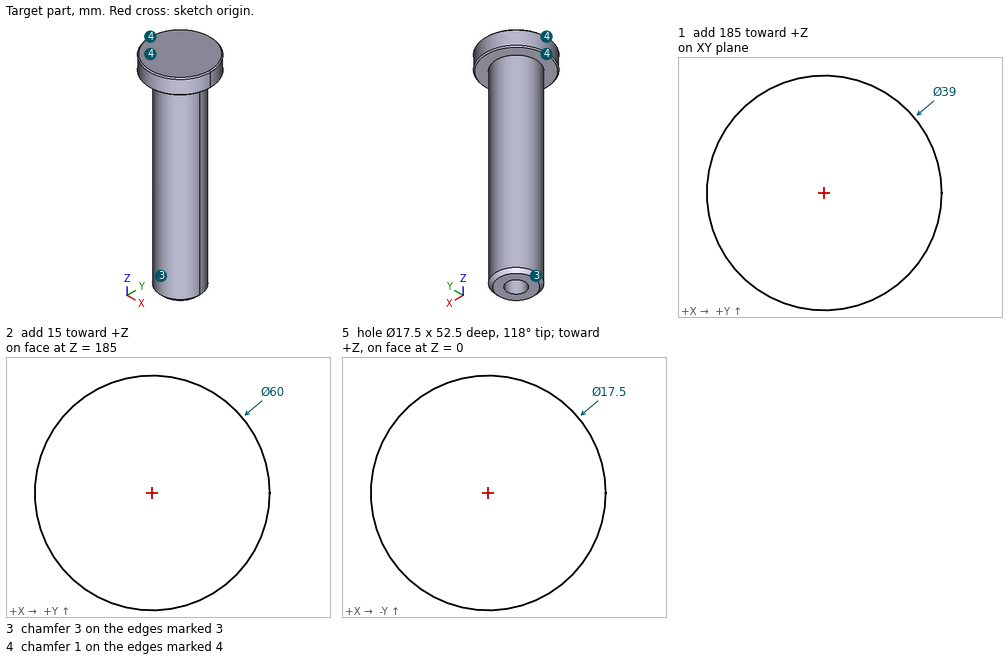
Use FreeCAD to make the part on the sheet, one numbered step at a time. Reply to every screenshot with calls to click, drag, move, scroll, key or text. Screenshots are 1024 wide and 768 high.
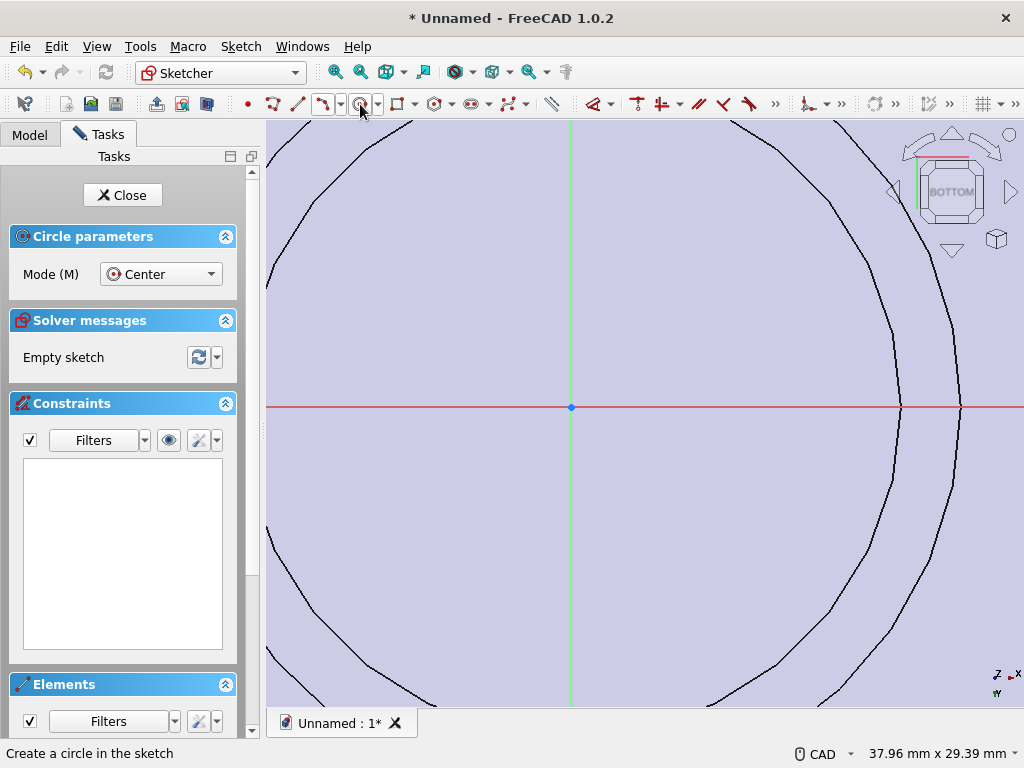
click(571, 407)
click(695, 284)
key(Escape)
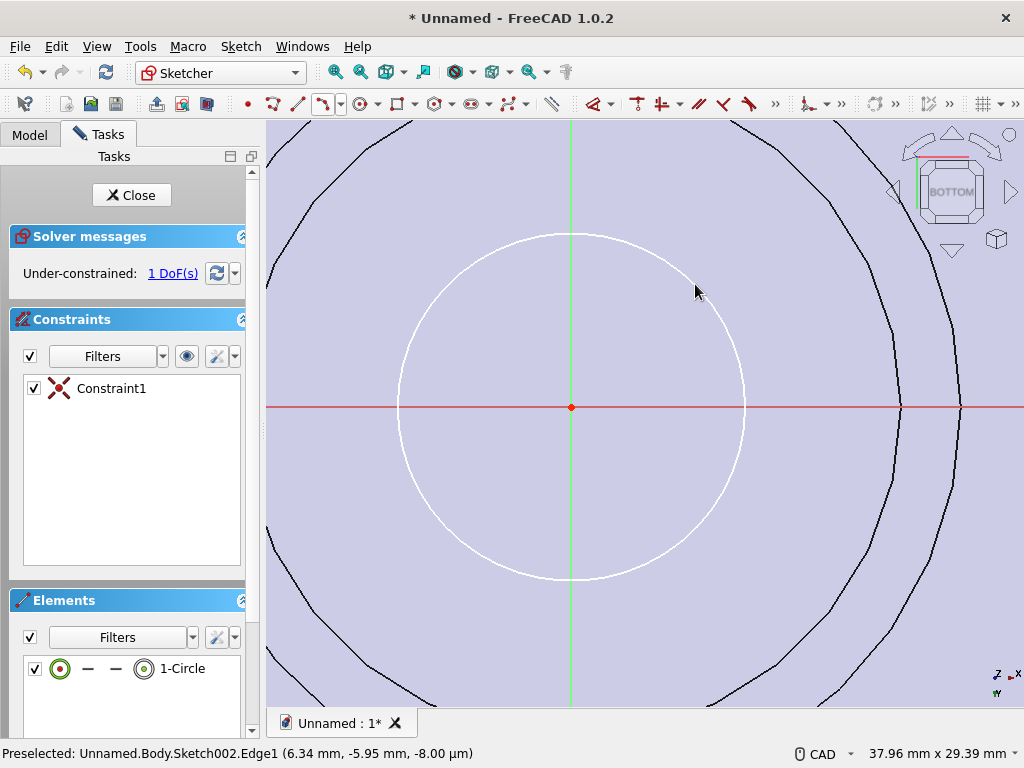
click(592, 104)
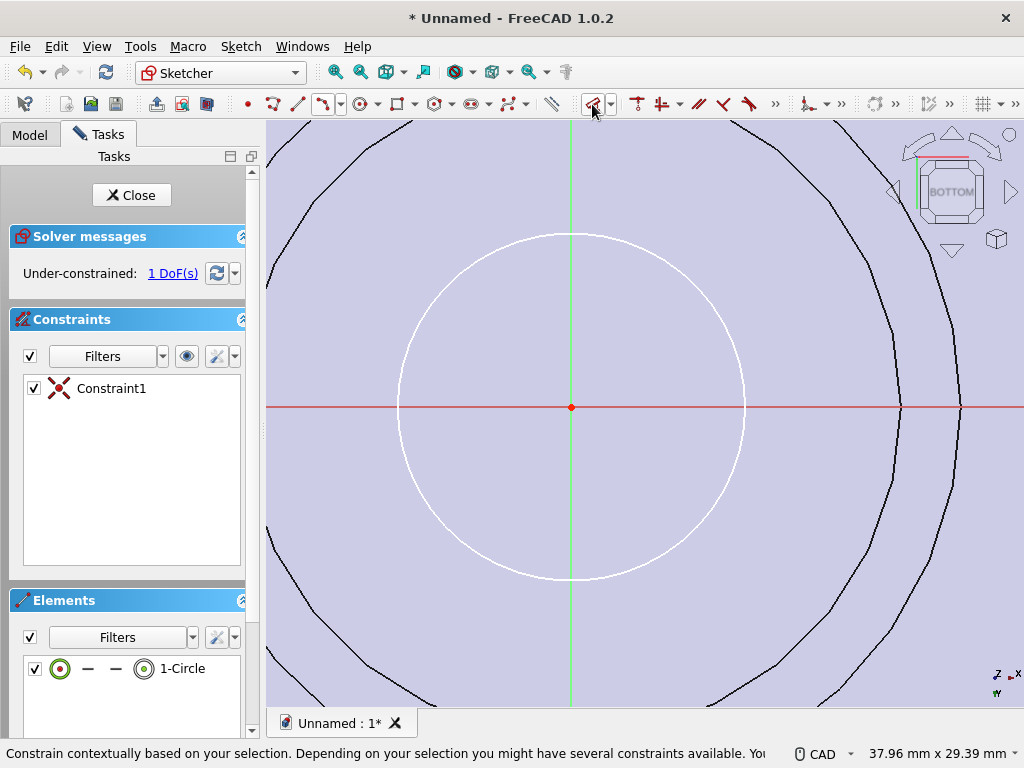
click(694, 284)
click(717, 261)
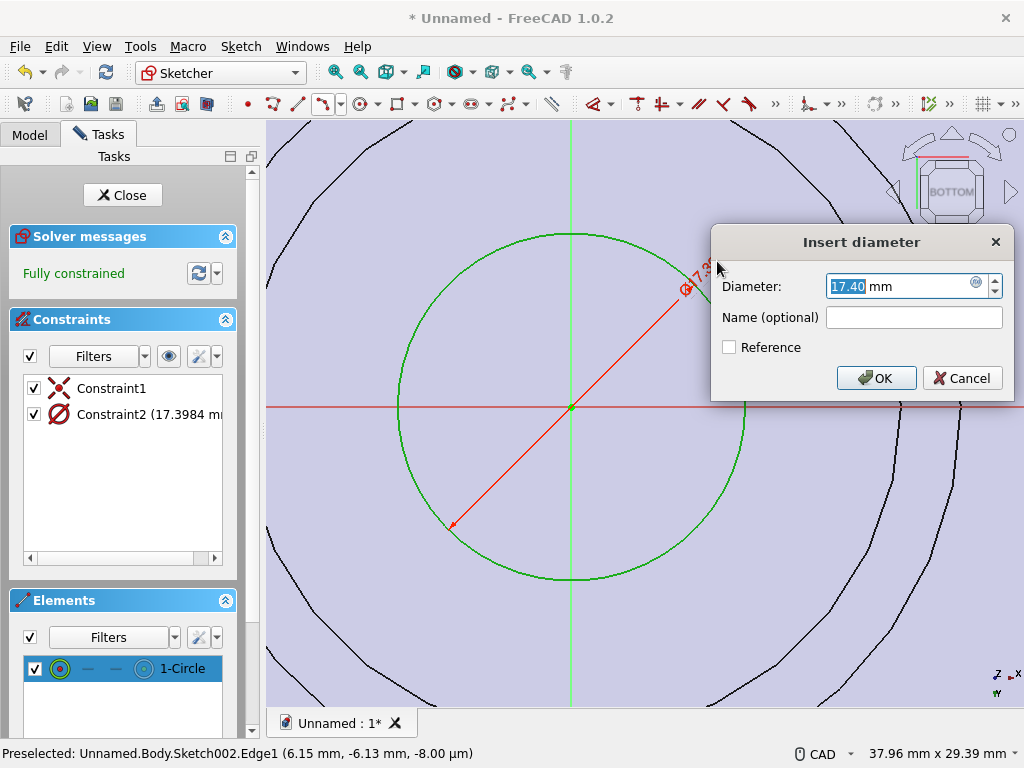
text(17.5)
key(Return)
key(Escape)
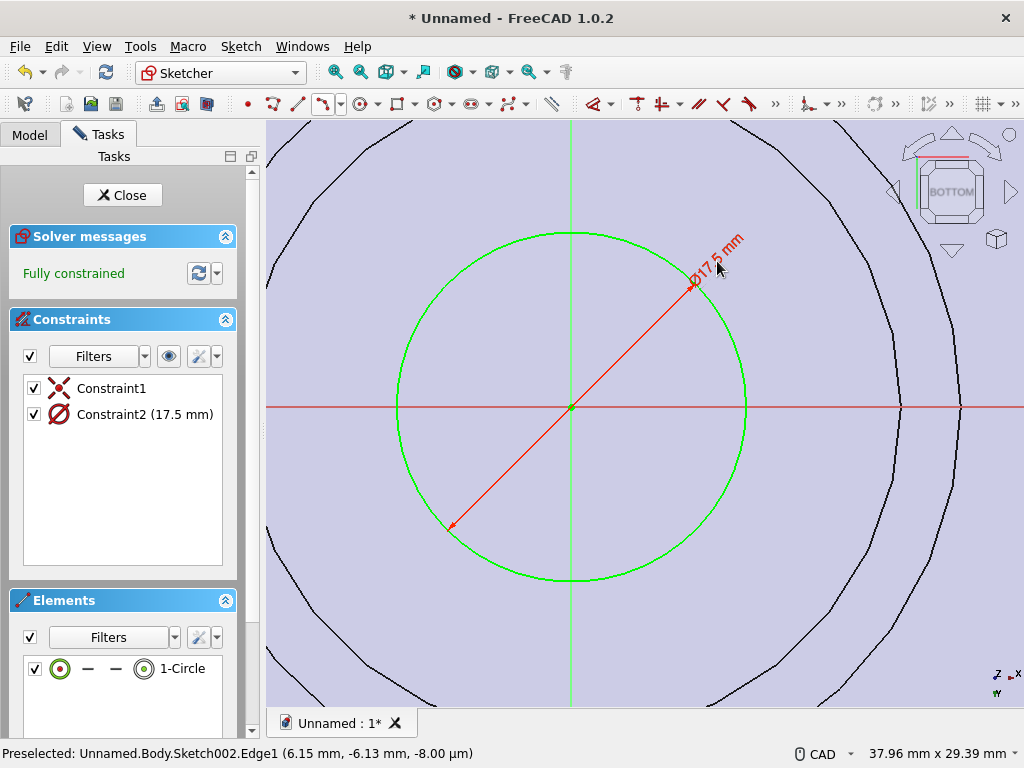
click(123, 195)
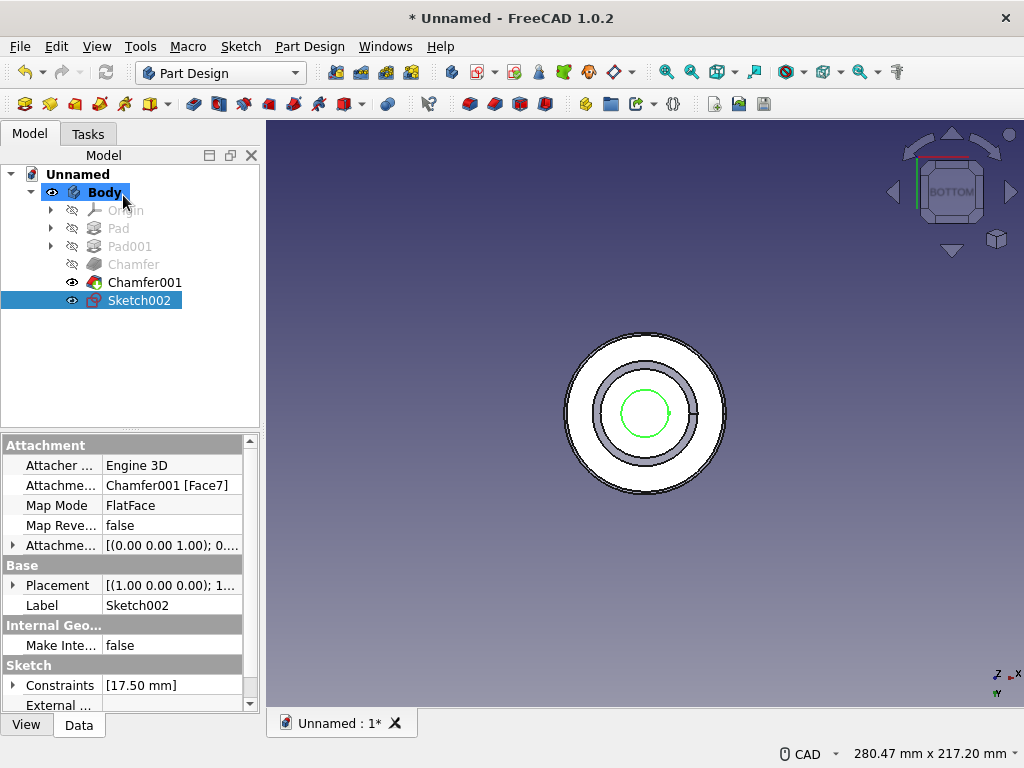
click(219, 104)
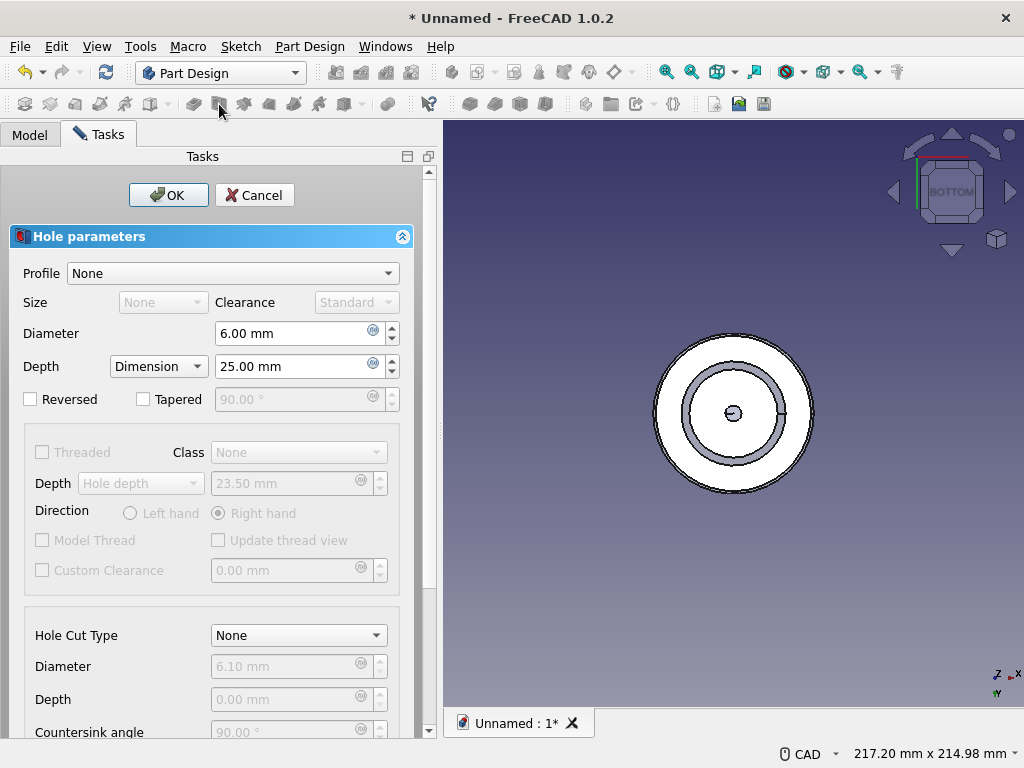
triple_click(300, 334)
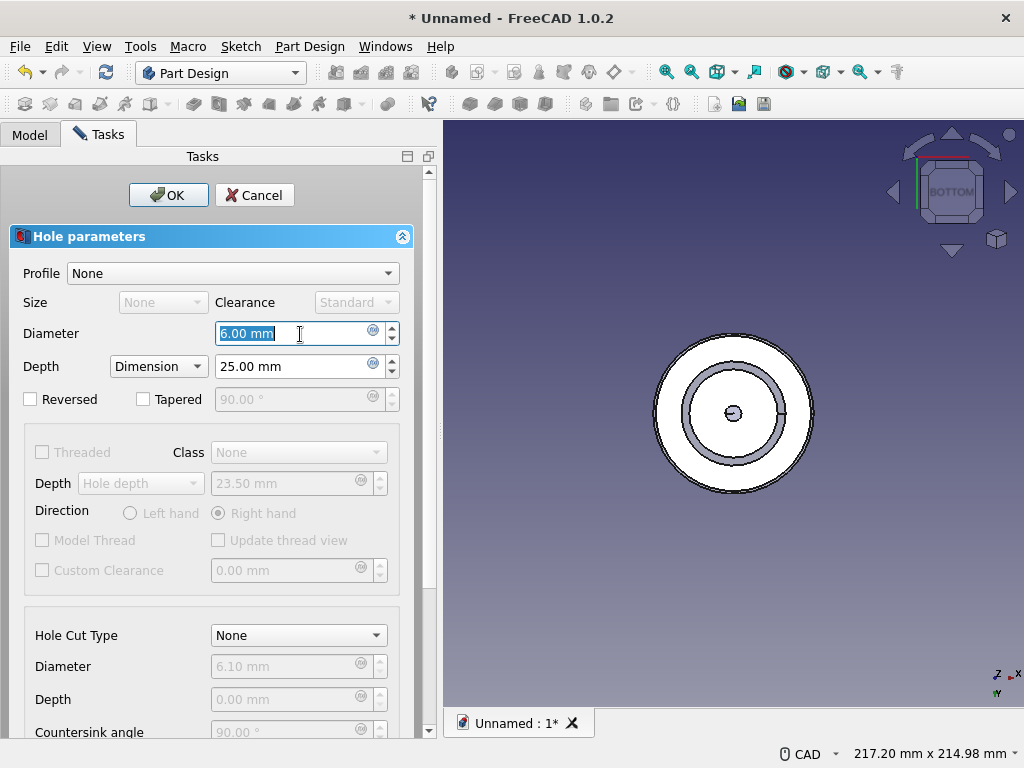
text(17.5)
key(Tab)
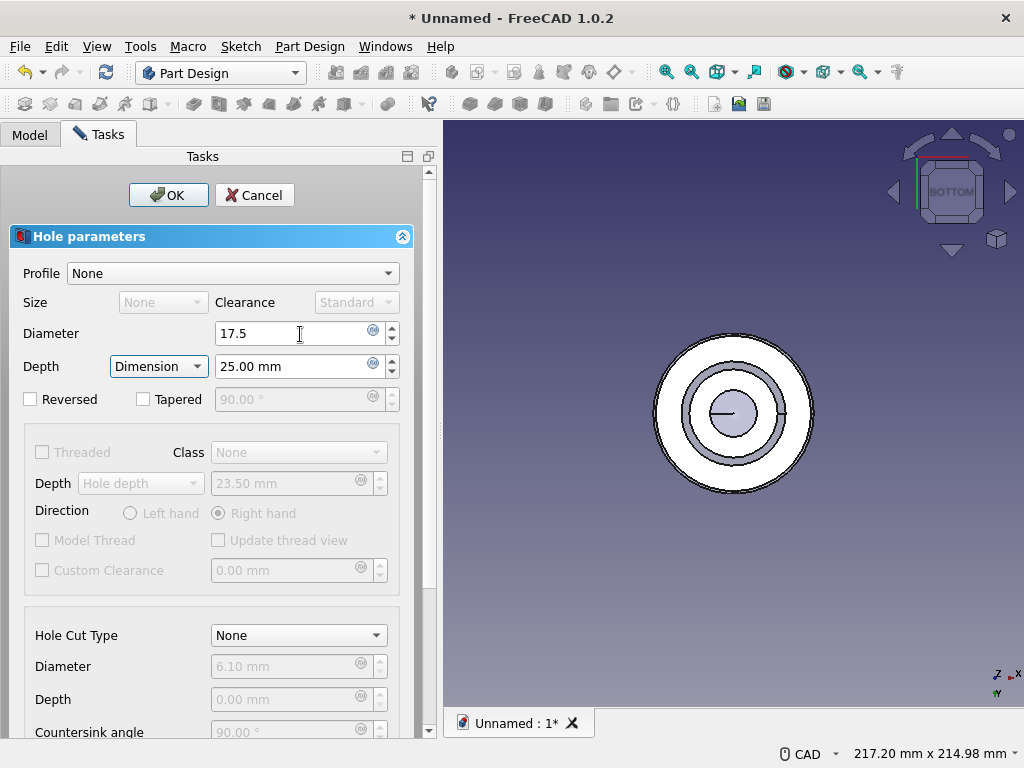
triple_click(300, 366)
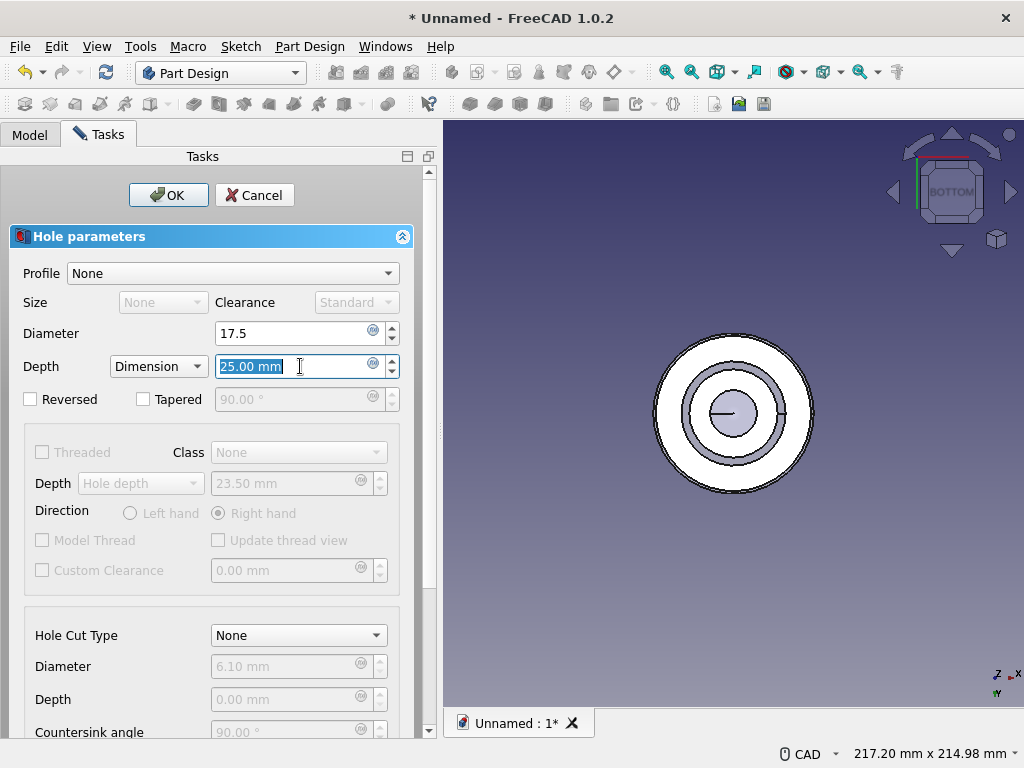
text(52.5)
key(Tab)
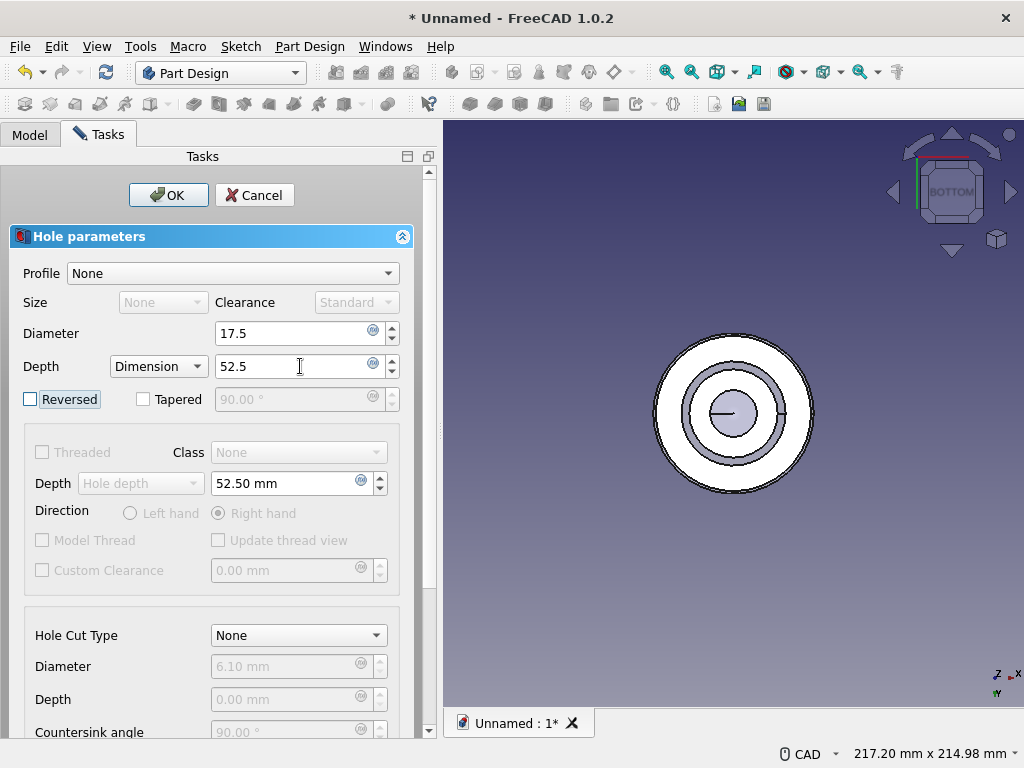
click(169, 195)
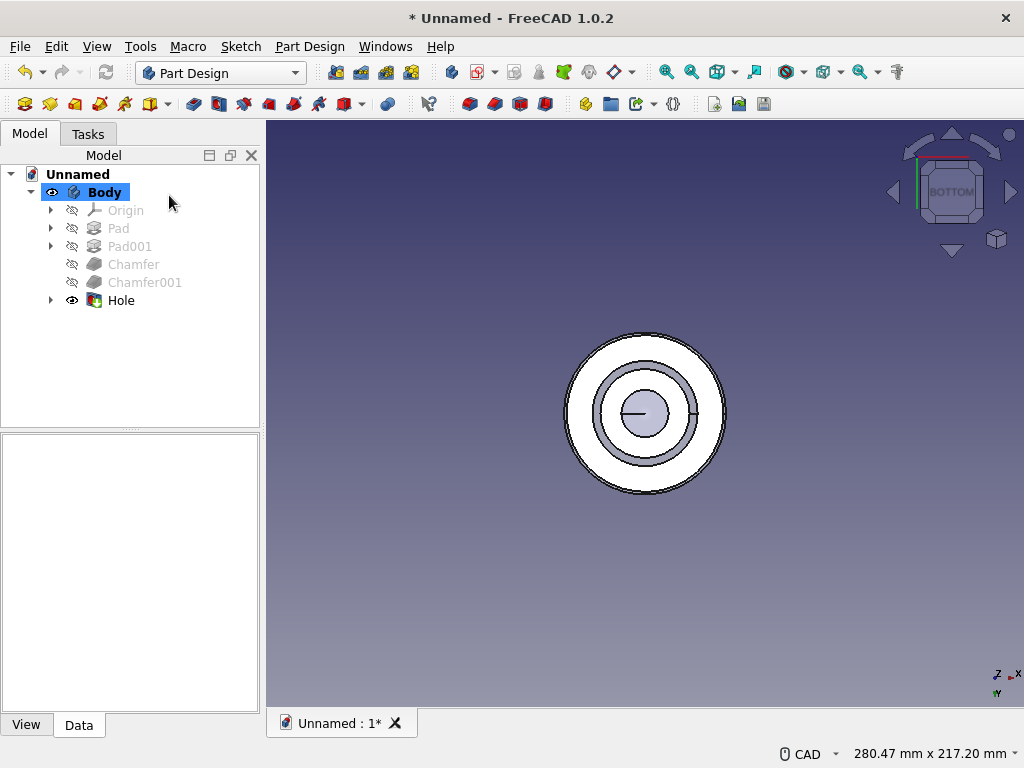
key(0)